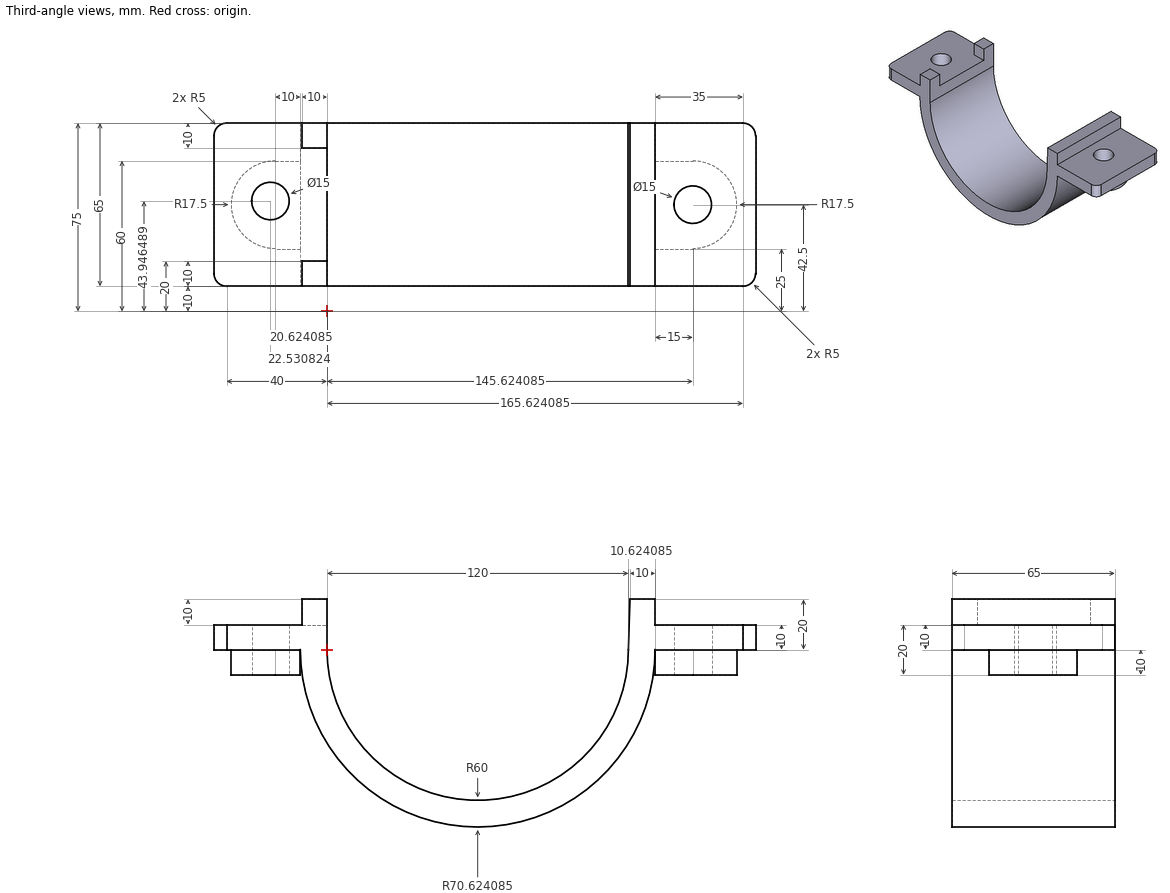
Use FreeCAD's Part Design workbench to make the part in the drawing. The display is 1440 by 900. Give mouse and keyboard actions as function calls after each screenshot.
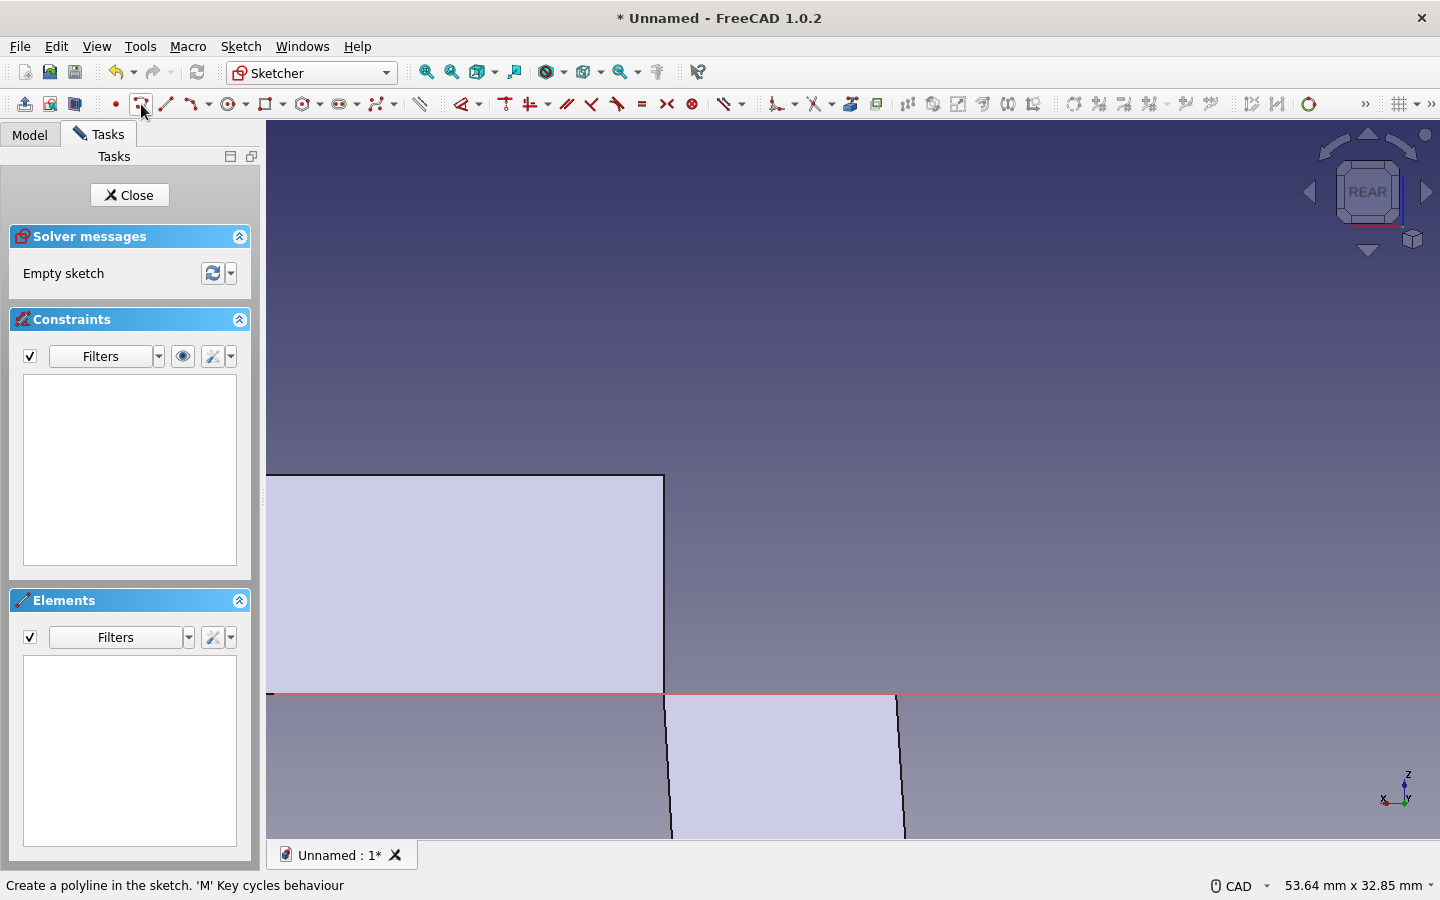
click(896, 694)
click(875, 257)
click(664, 257)
click(664, 685)
click(896, 694)
key(Escape)
key(Escape)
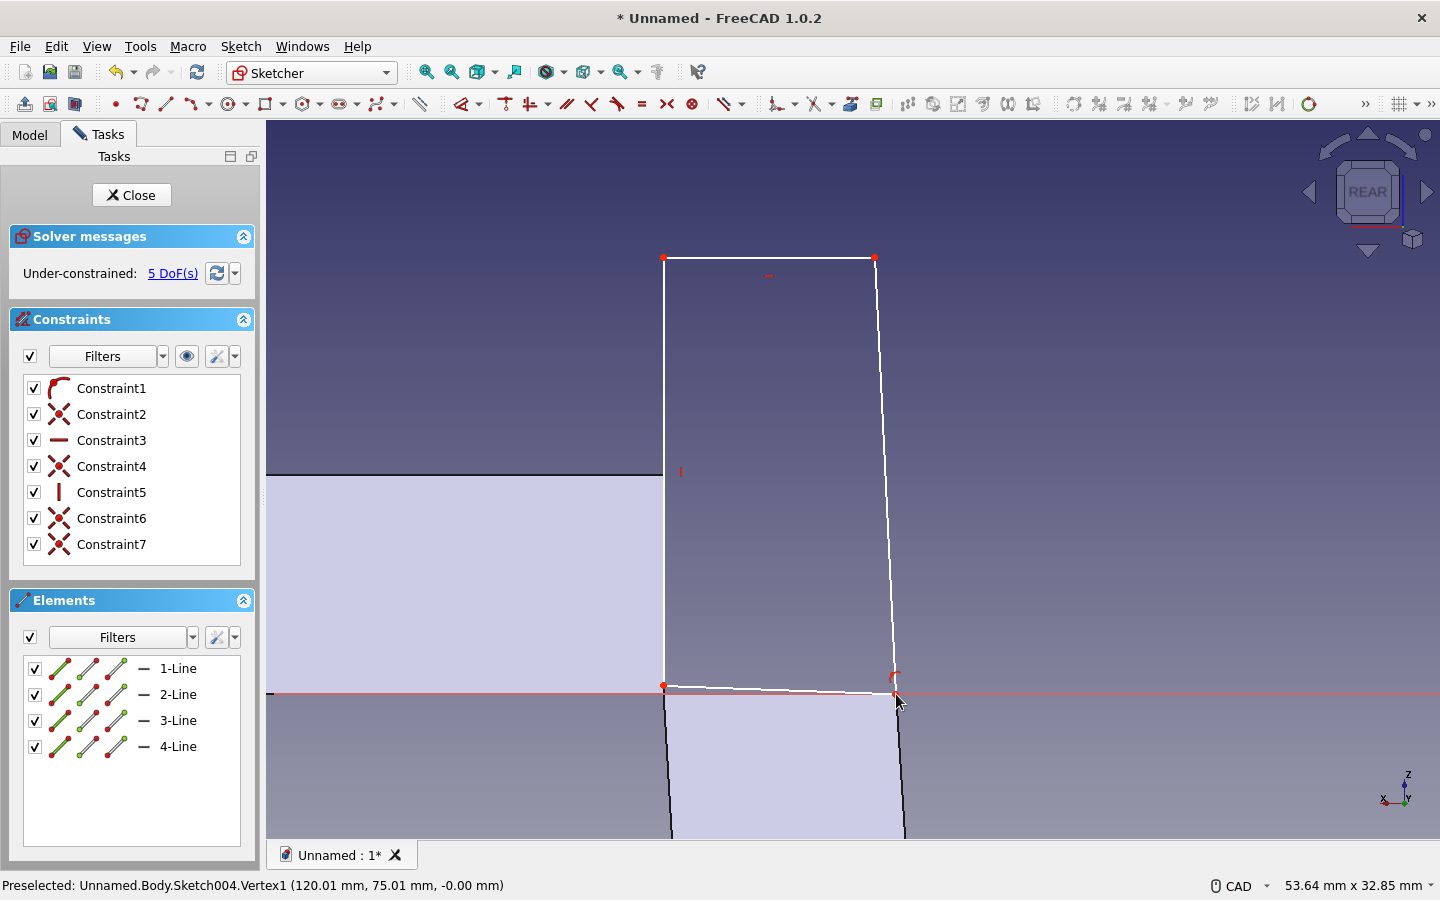
click(826, 692)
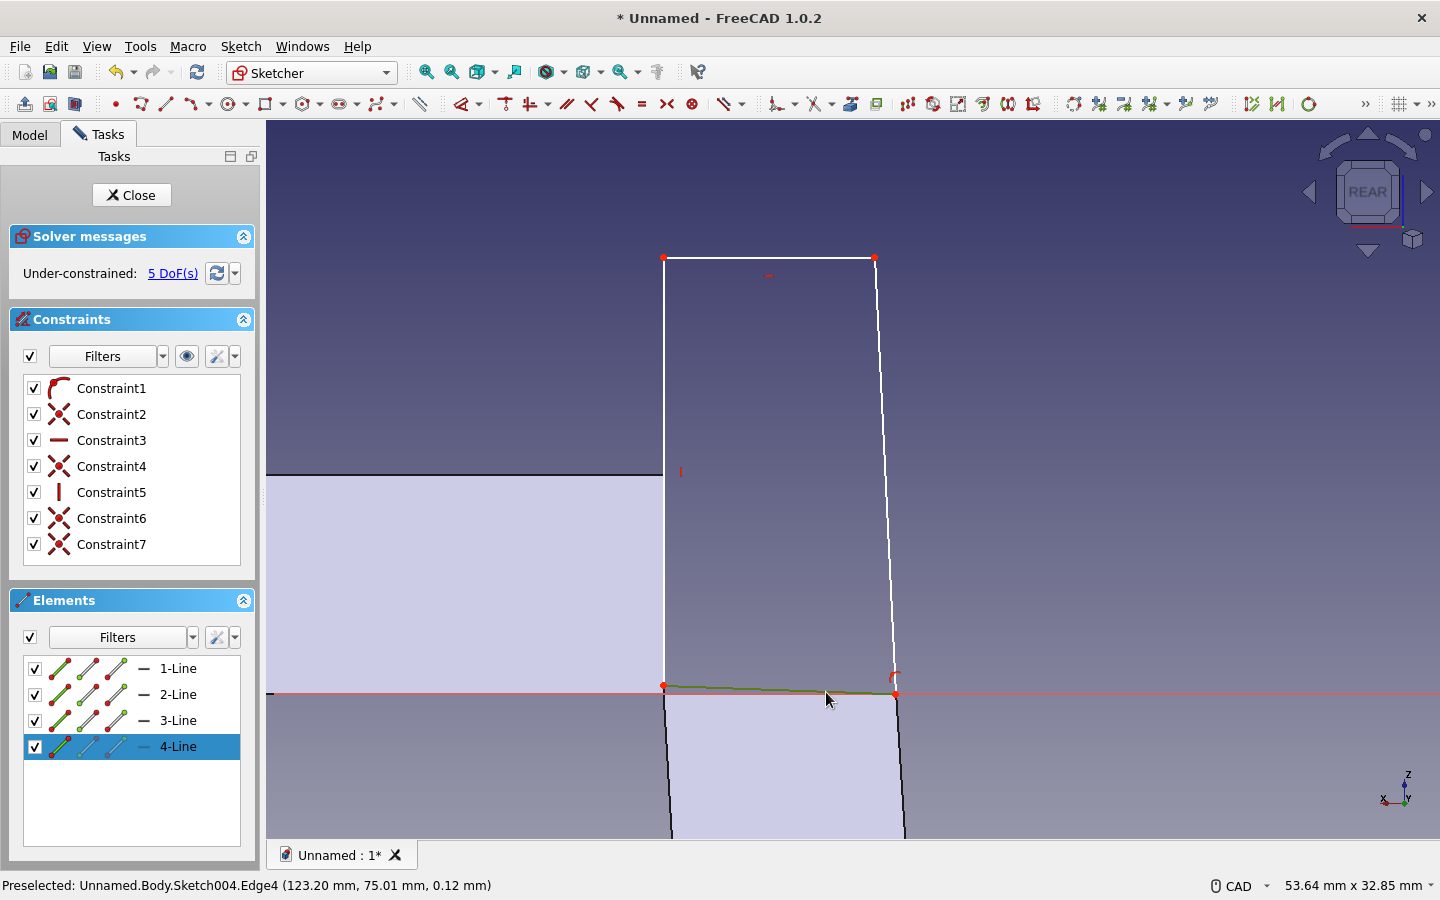
key(h)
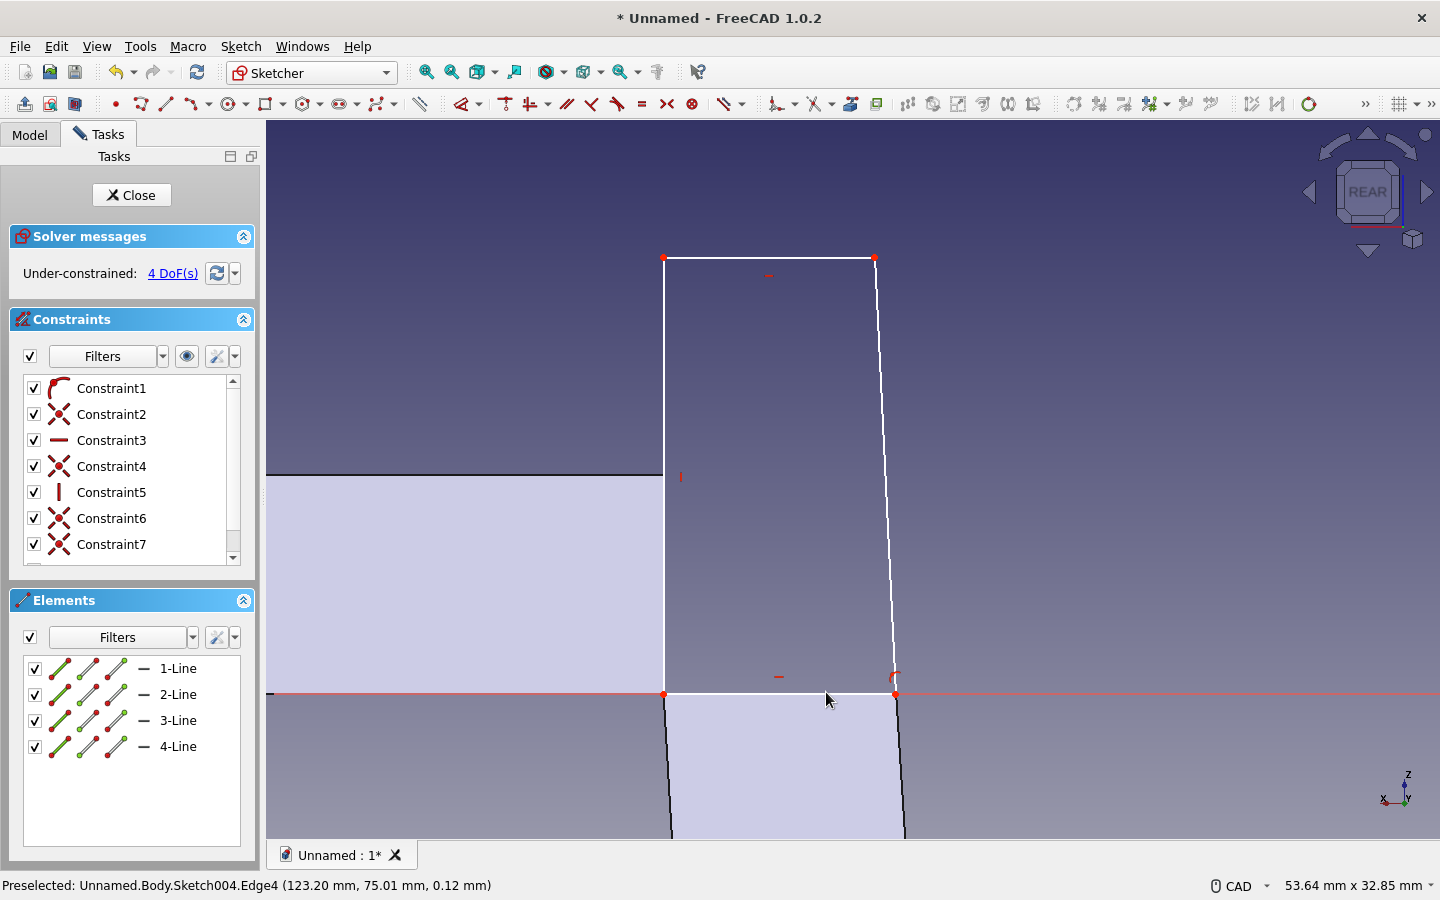
key(d)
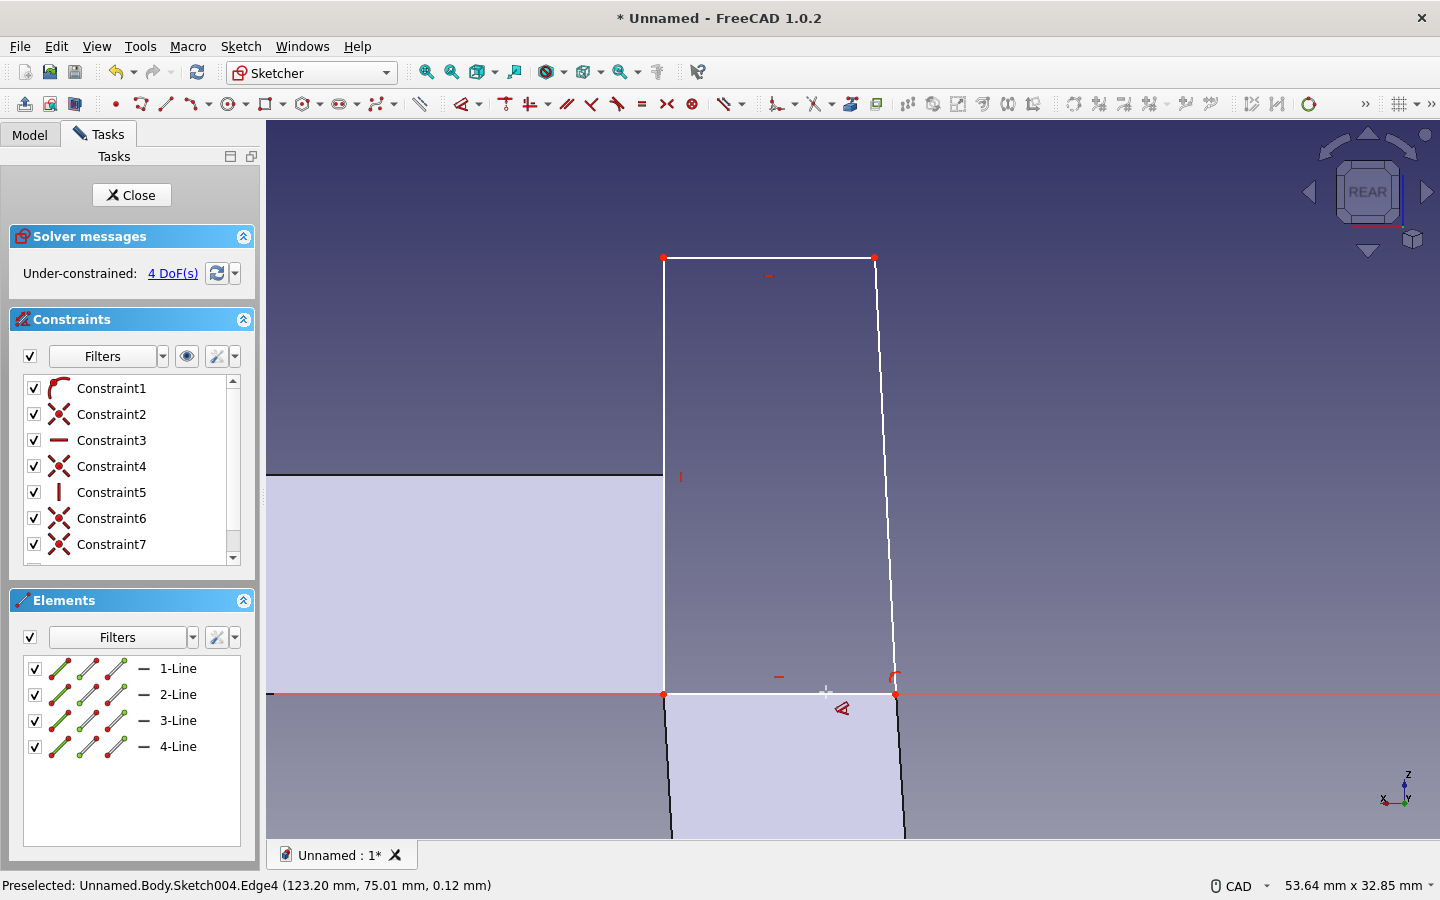
click(812, 258)
click(770, 224)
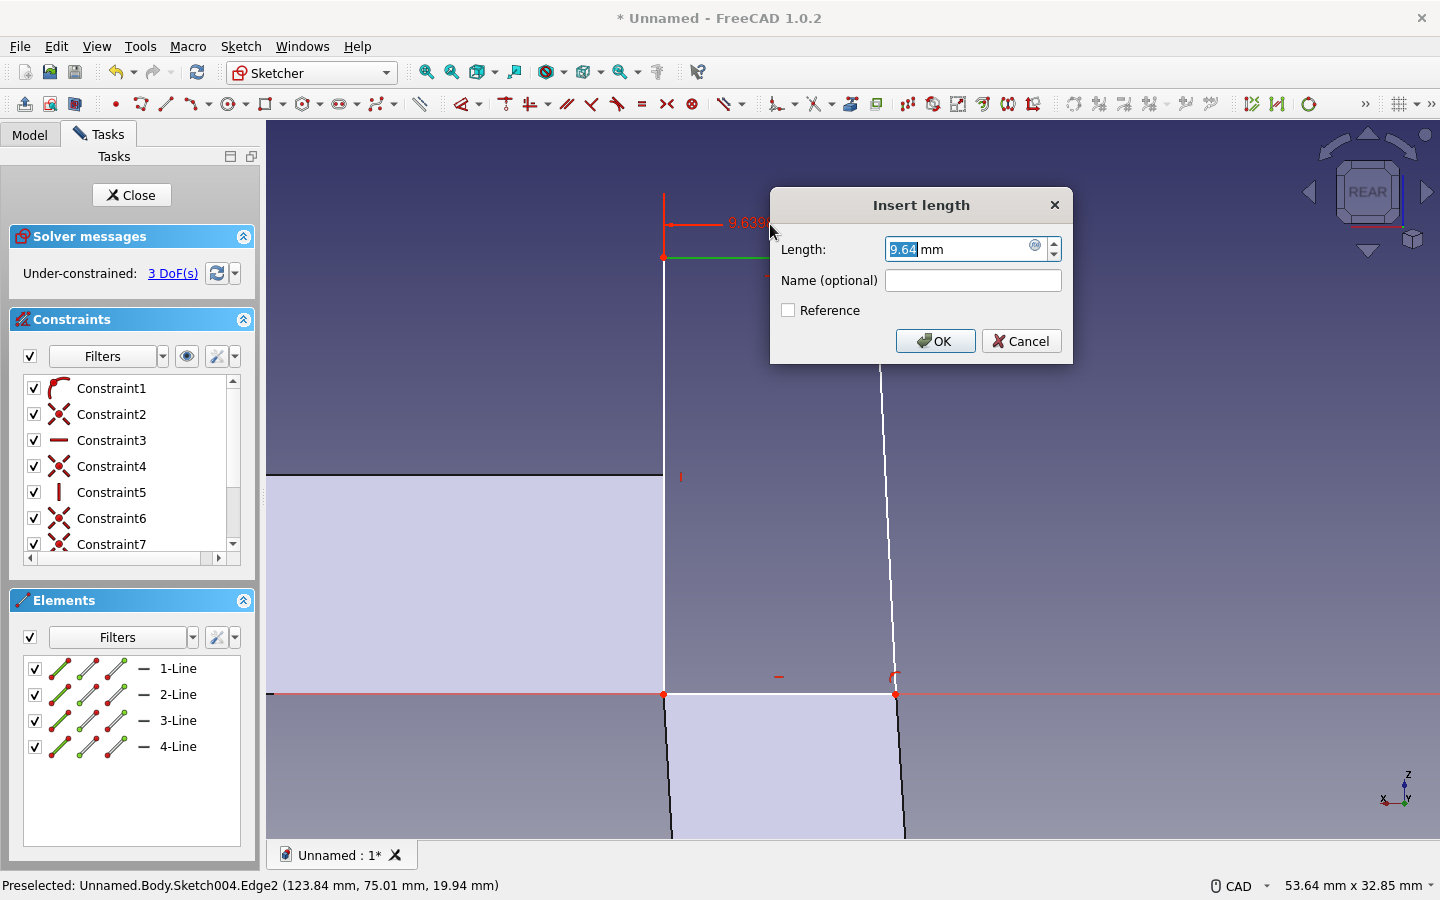
text(10)
key(Return)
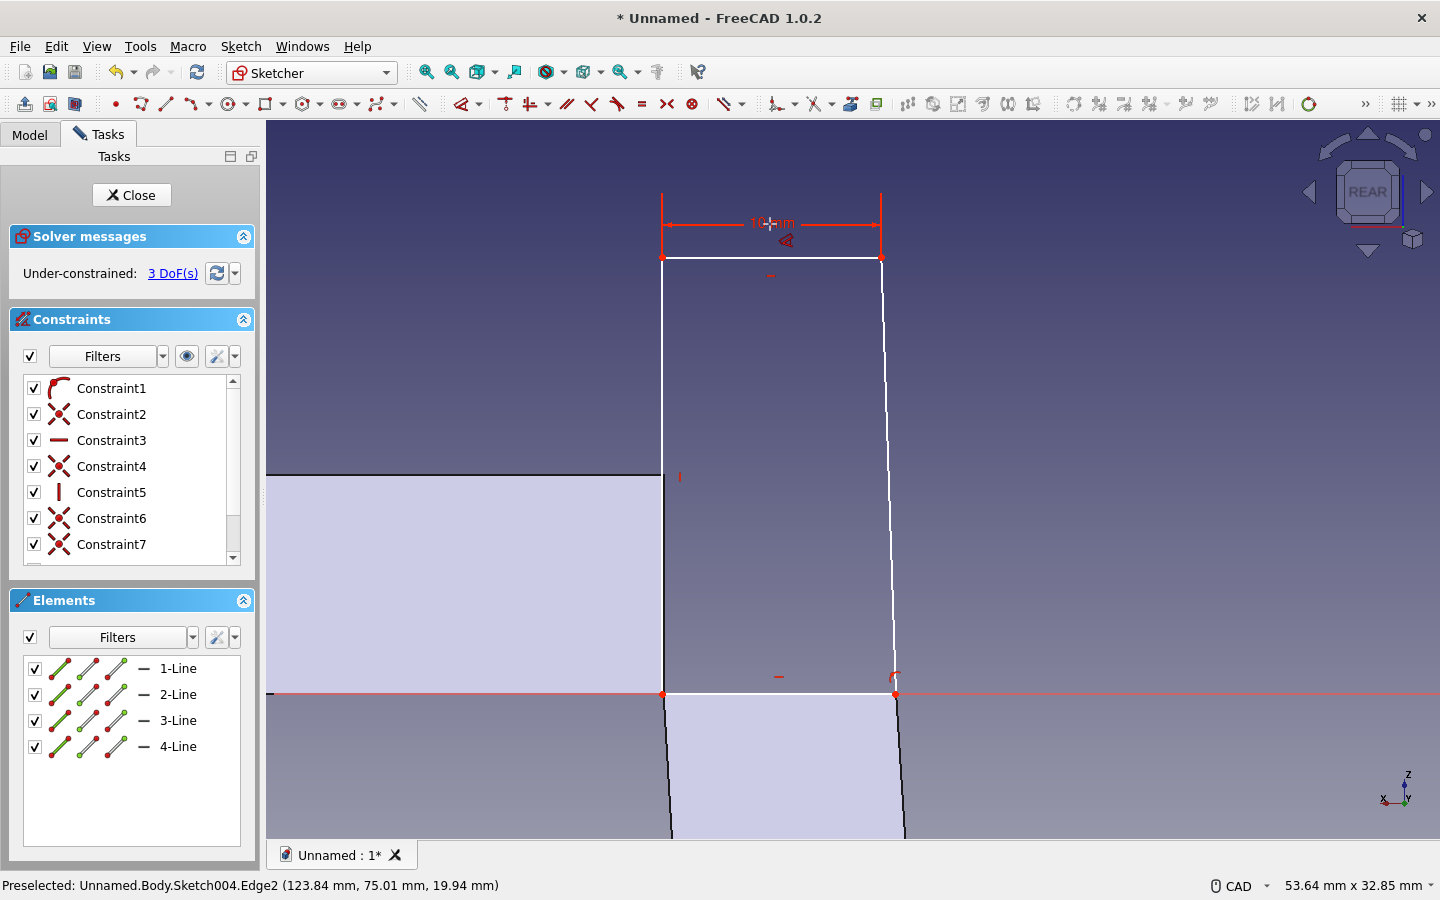
click(662, 389)
click(628, 476)